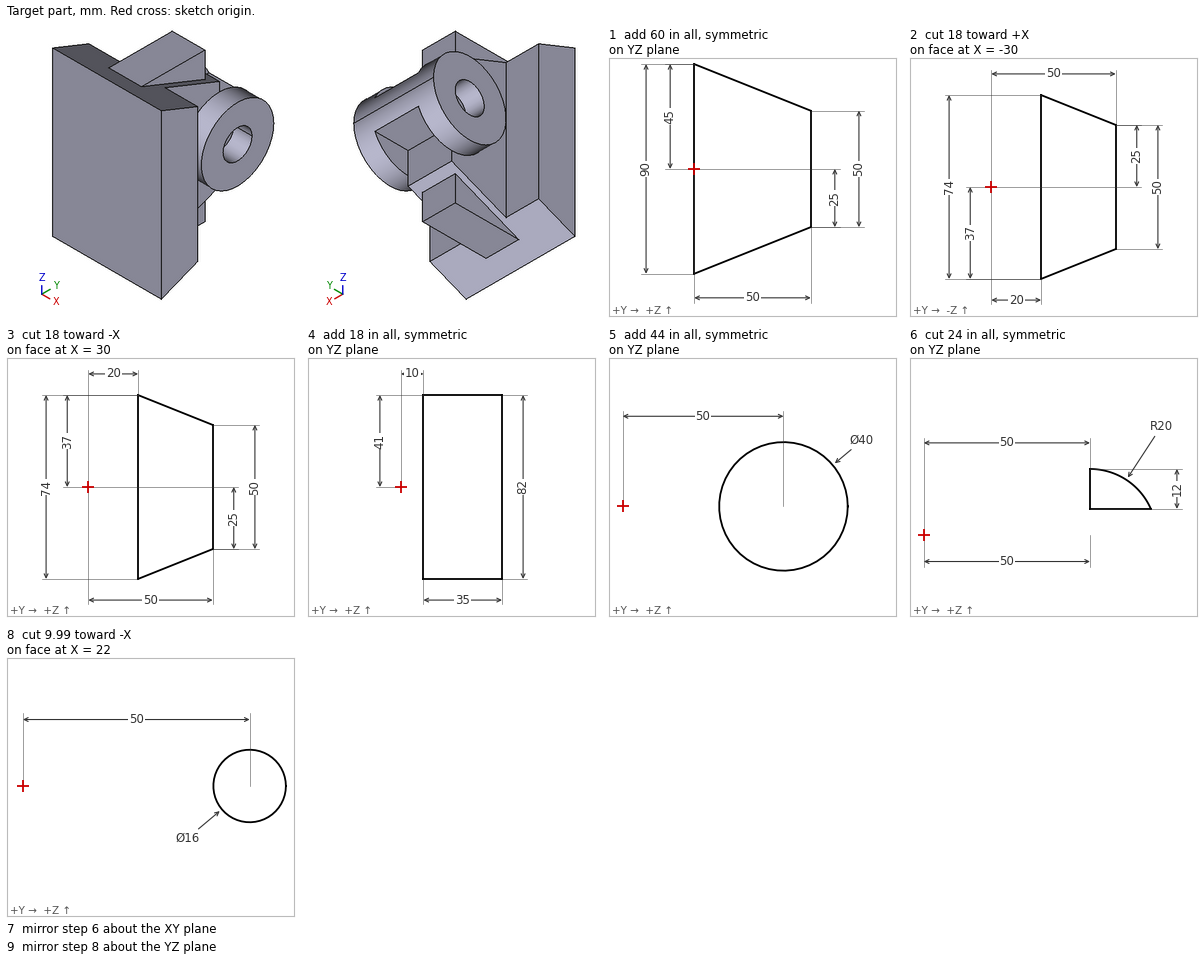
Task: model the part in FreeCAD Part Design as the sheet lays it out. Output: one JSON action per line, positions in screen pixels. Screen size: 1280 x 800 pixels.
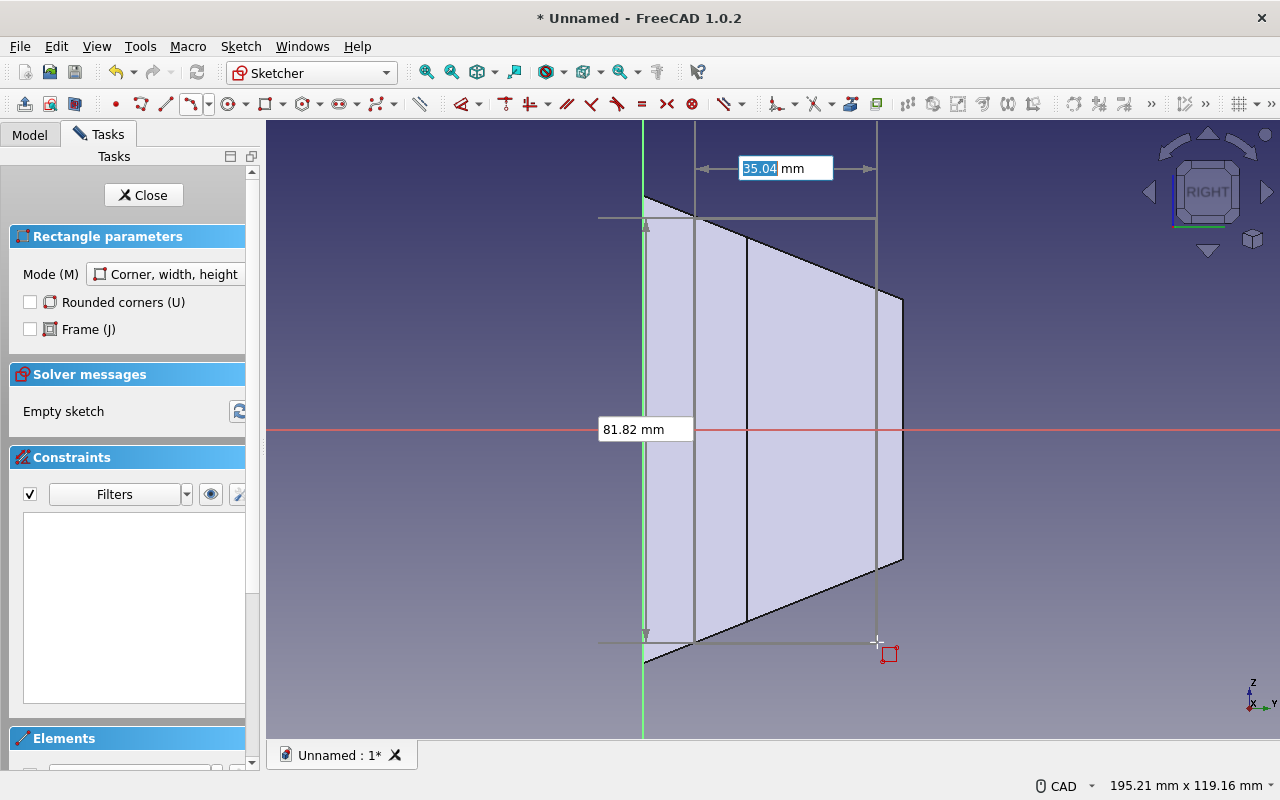
{"action": "type", "text": "35"}
{"action": "key", "text": "Tab"}
{"action": "type", "text": "82"}
{"action": "key", "text": "Return"}
{"action": "key", "text": "Escape"}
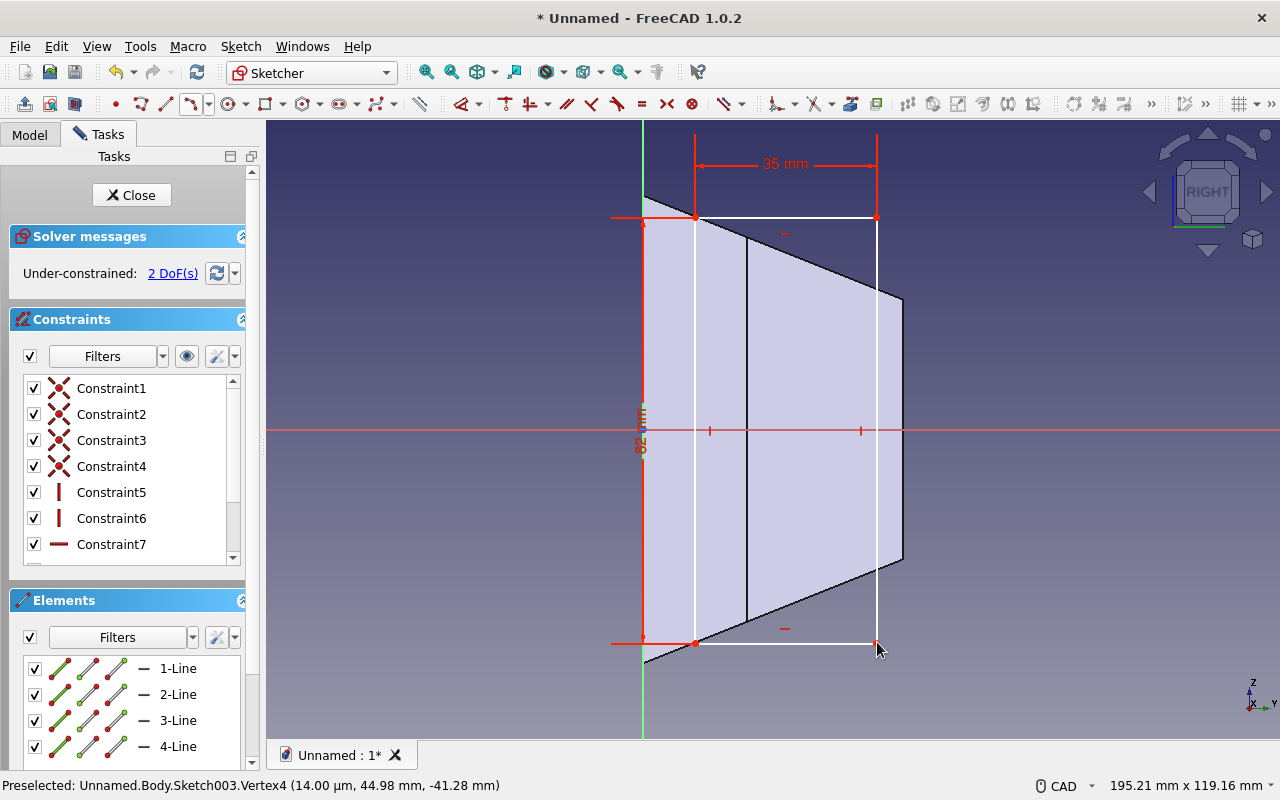
{"action": "left_click", "coordinate": [460, 104]}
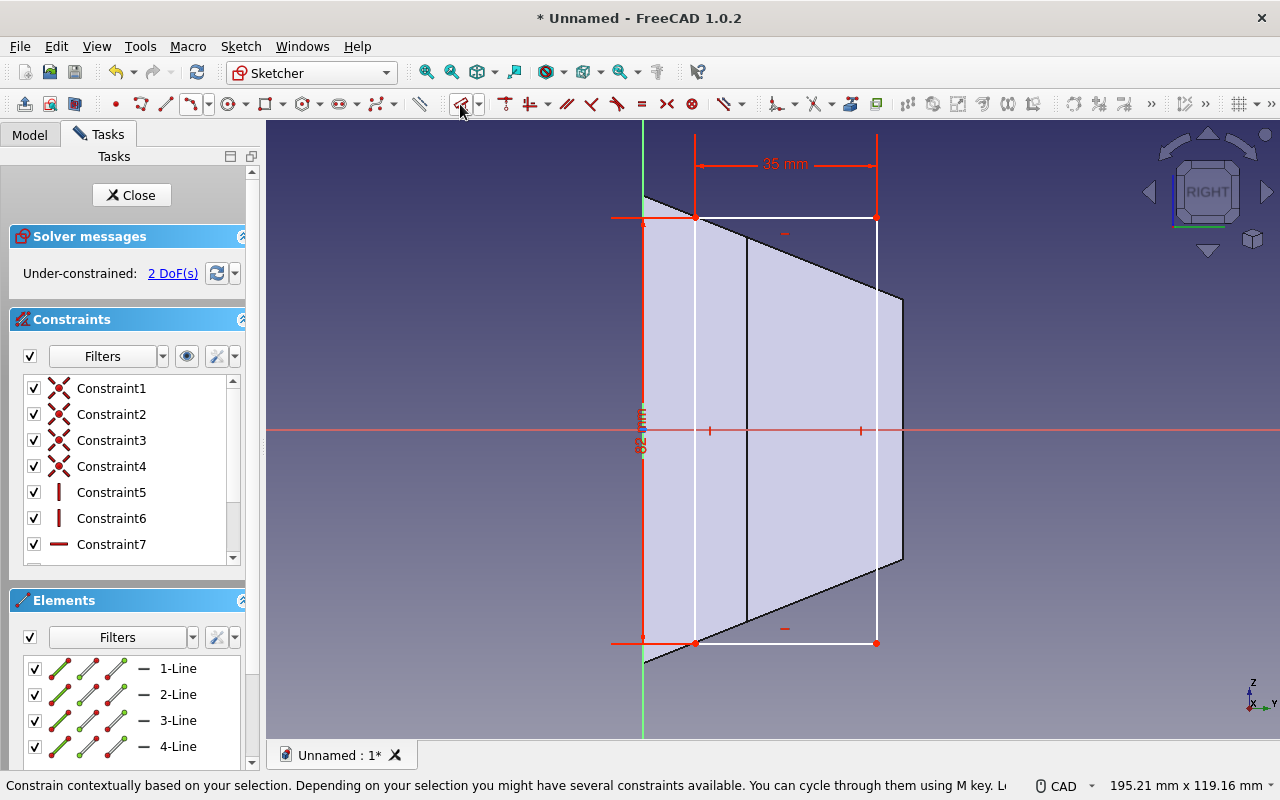
{"action": "left_click", "coordinate": [695, 218]}
{"action": "left_click", "coordinate": [669, 184]}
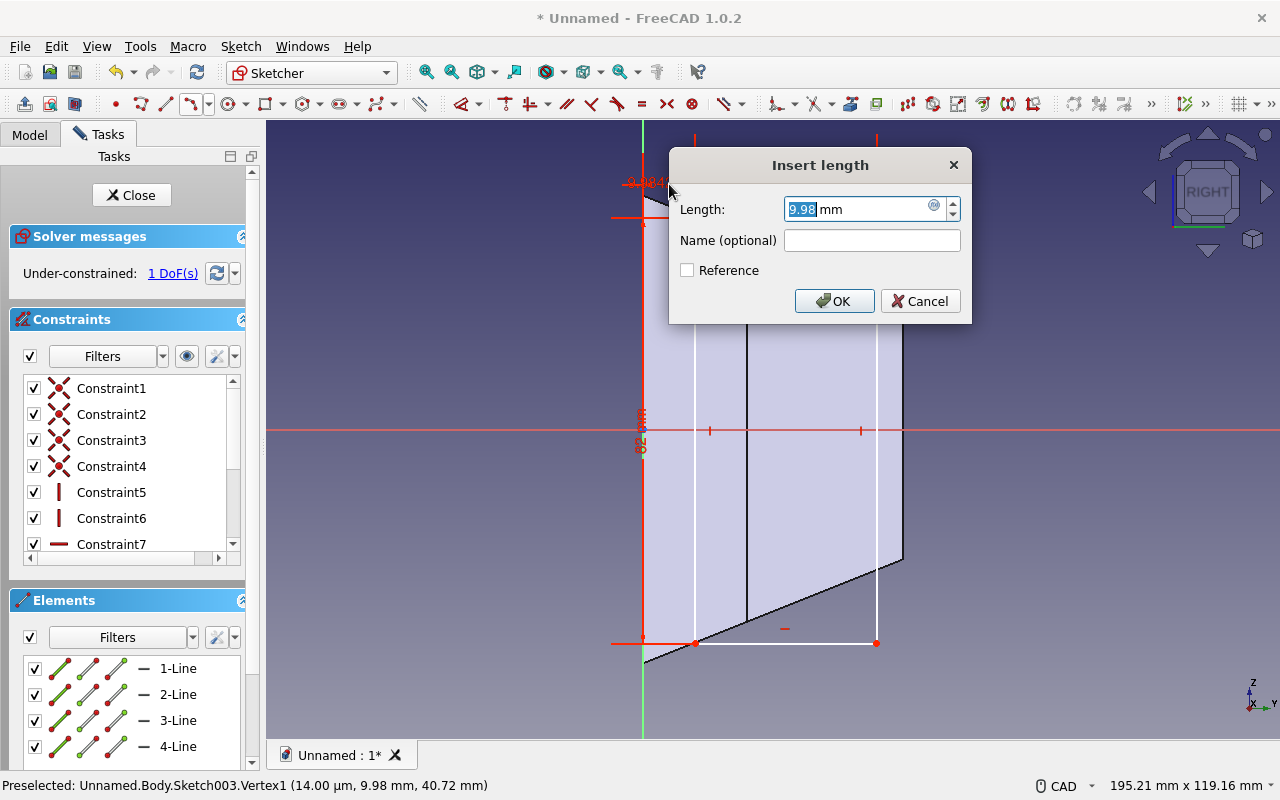
{"action": "type", "text": "10"}
{"action": "key", "text": "Return"}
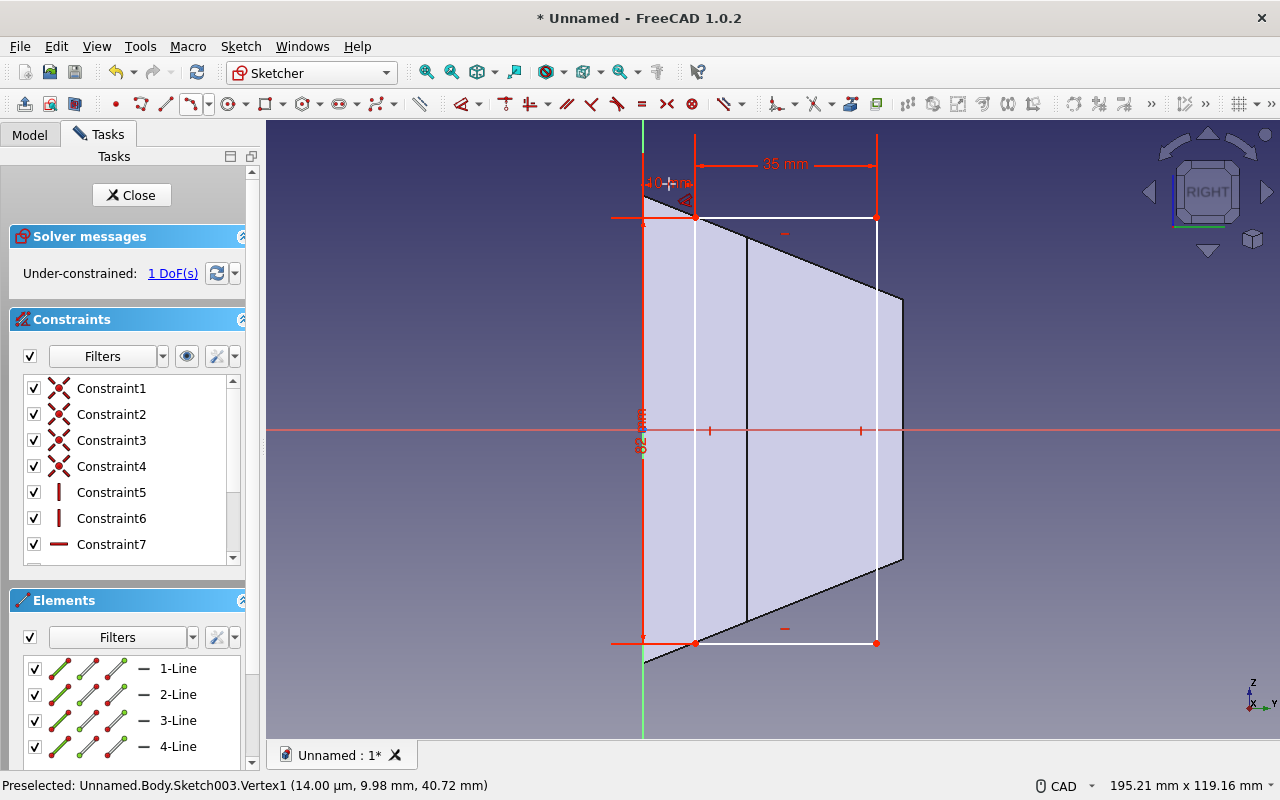
{"action": "left_click", "coordinate": [695, 218]}
{"action": "left_click", "coordinate": [609, 324]}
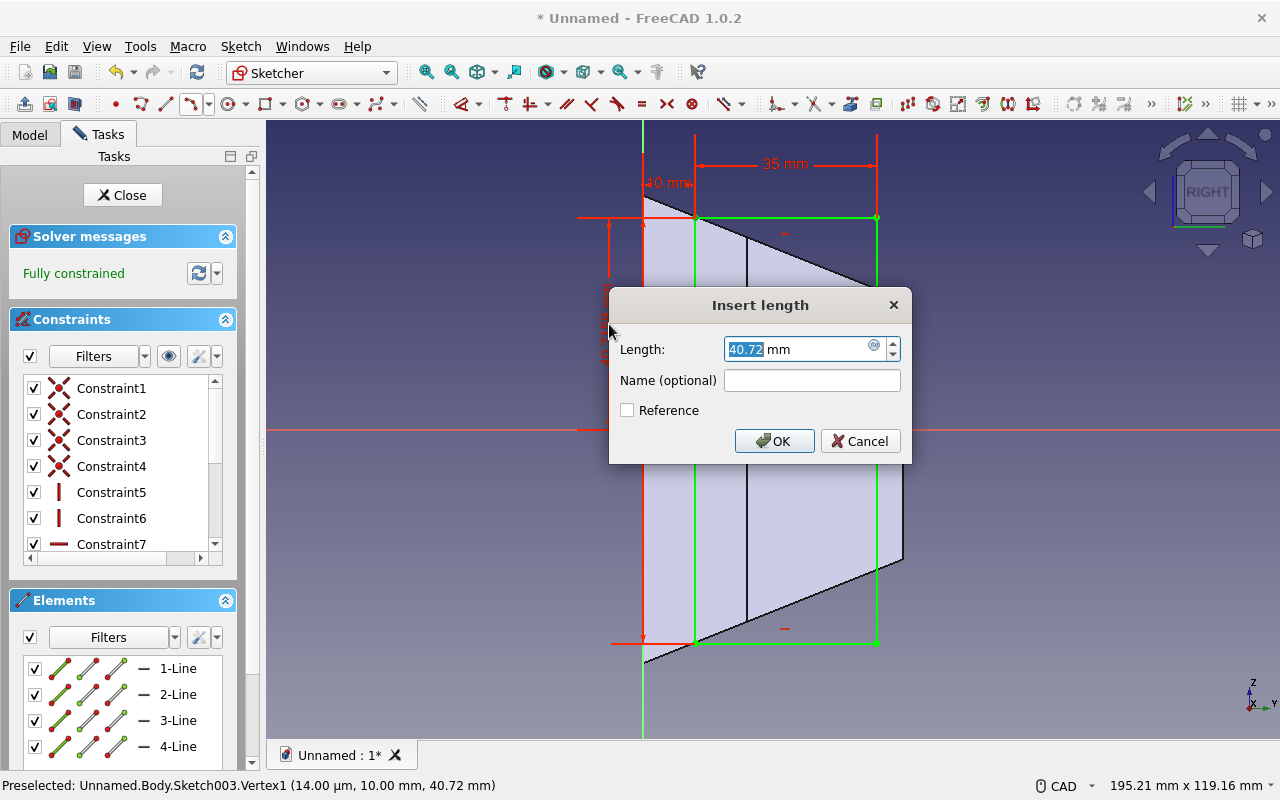
{"action": "type", "text": "41"}
{"action": "key", "text": "Return"}
{"action": "key", "text": "Escape"}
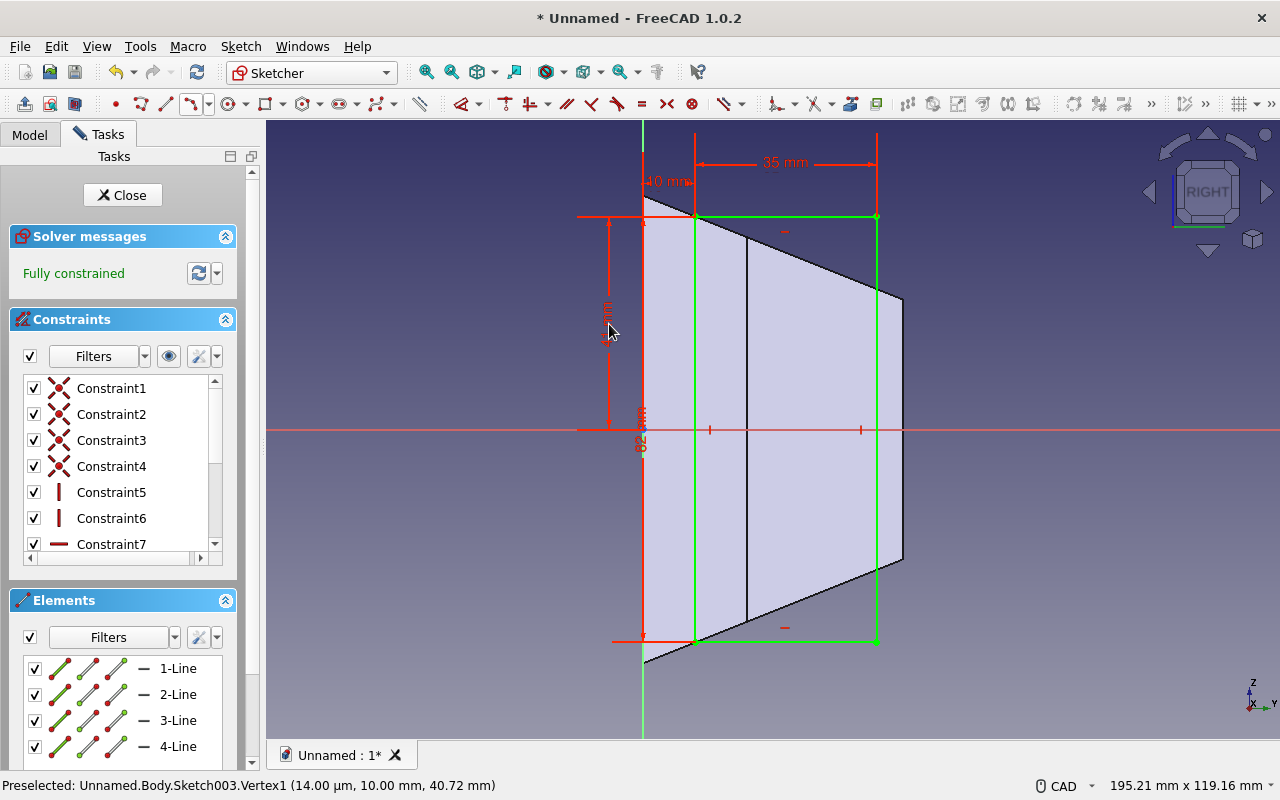
{"action": "left_click", "coordinate": [123, 195]}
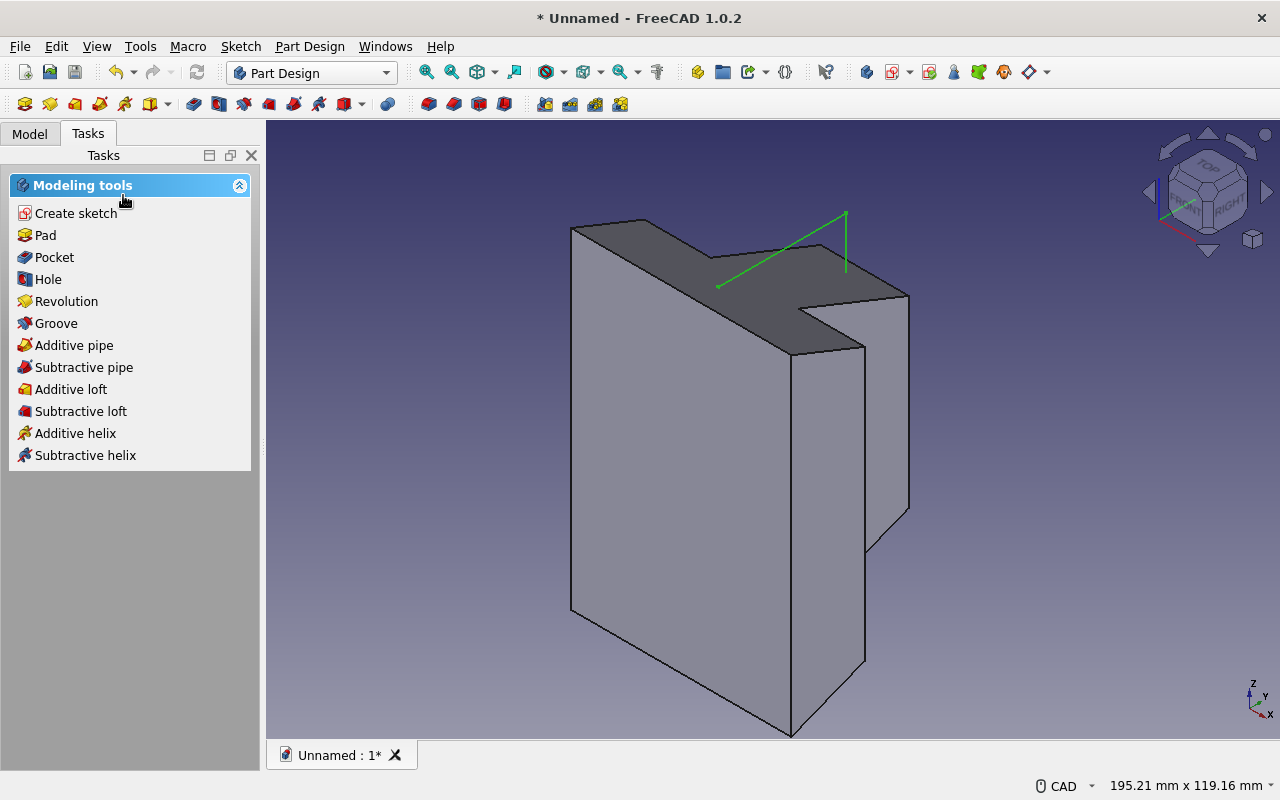
{"action": "left_click", "coordinate": [25, 104]}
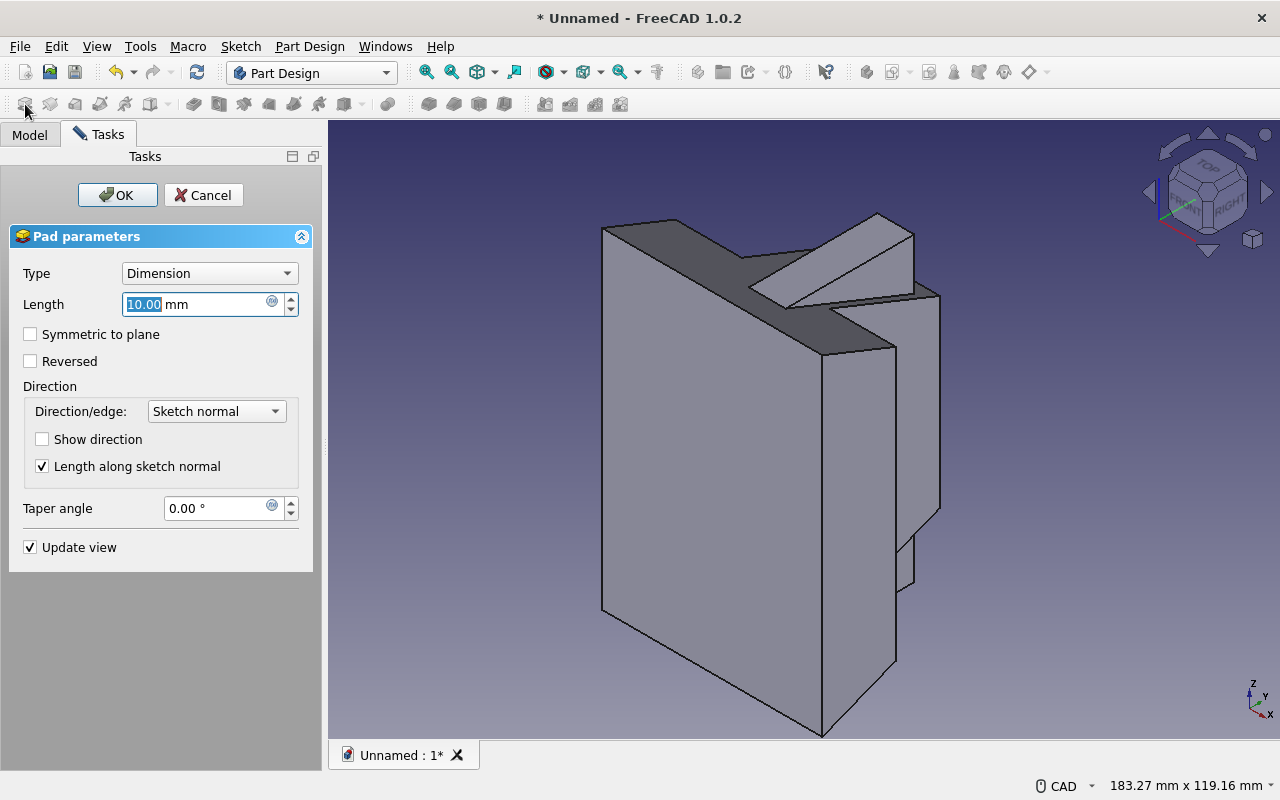
{"action": "type", "text": "18"}
{"action": "key", "text": "Tab"}